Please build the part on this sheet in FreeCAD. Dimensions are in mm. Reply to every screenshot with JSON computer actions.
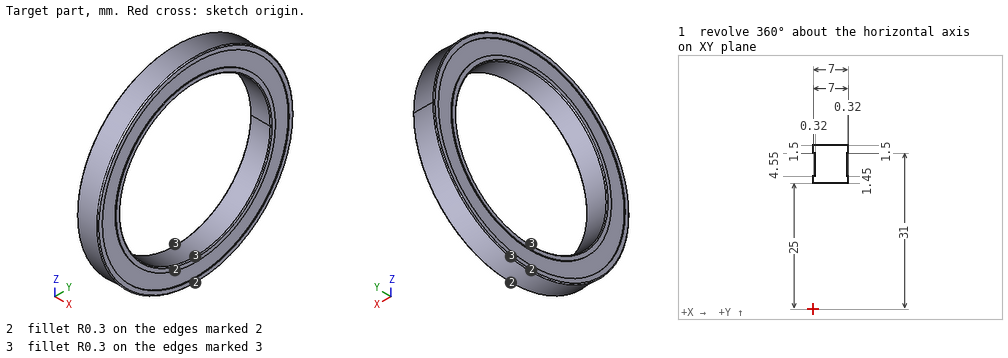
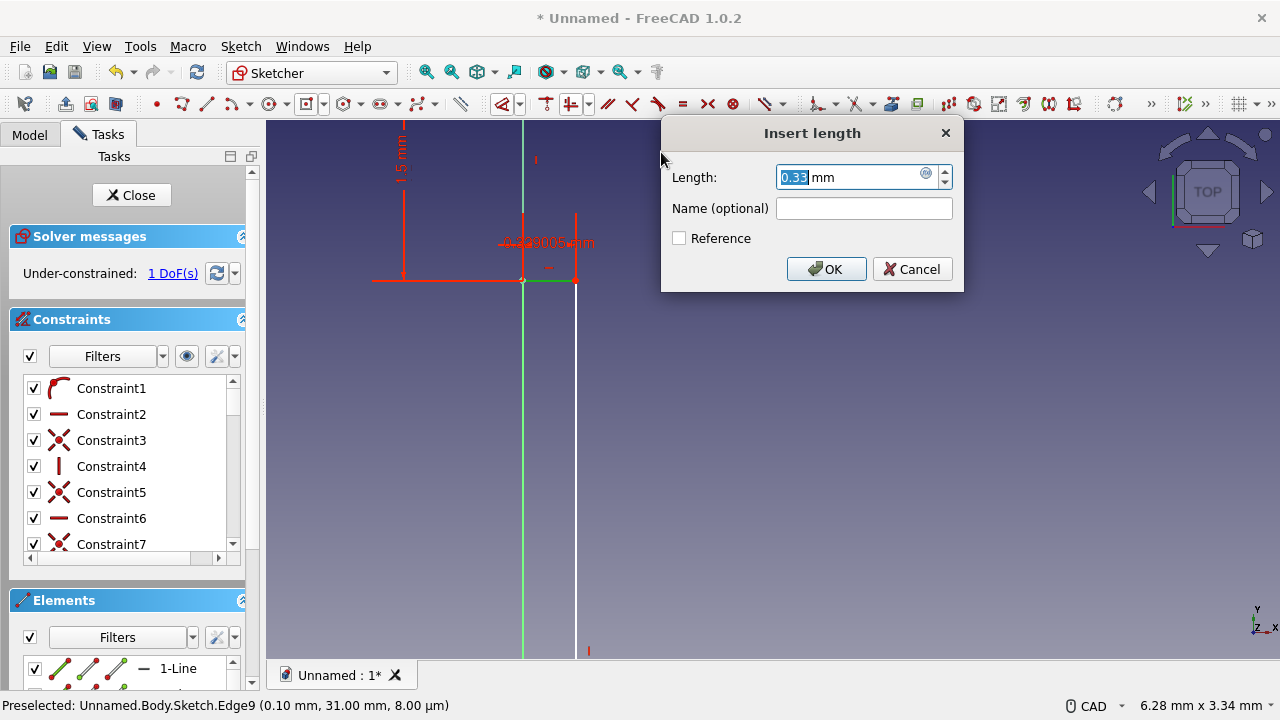
{"action": "type", "text": "0.32"}
{"action": "key", "text": "Return"}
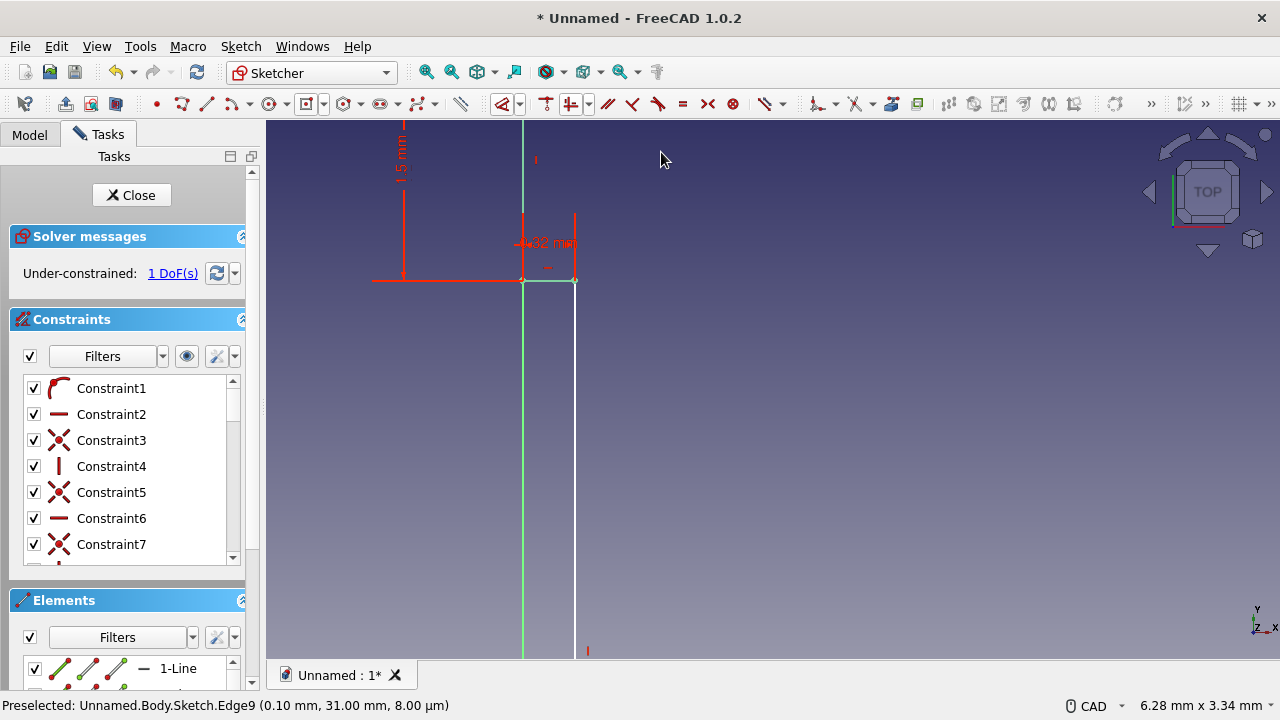
{"action": "left_click", "coordinate": [575, 502]}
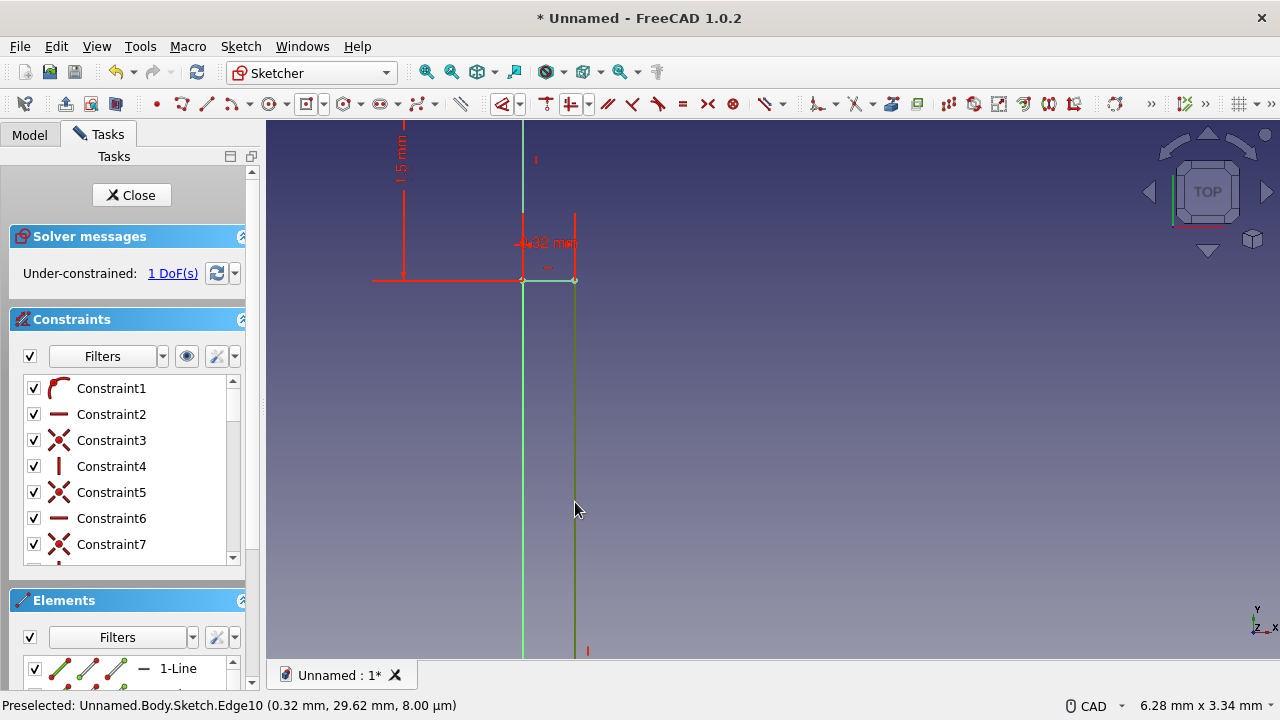
{"action": "key", "text": "i"}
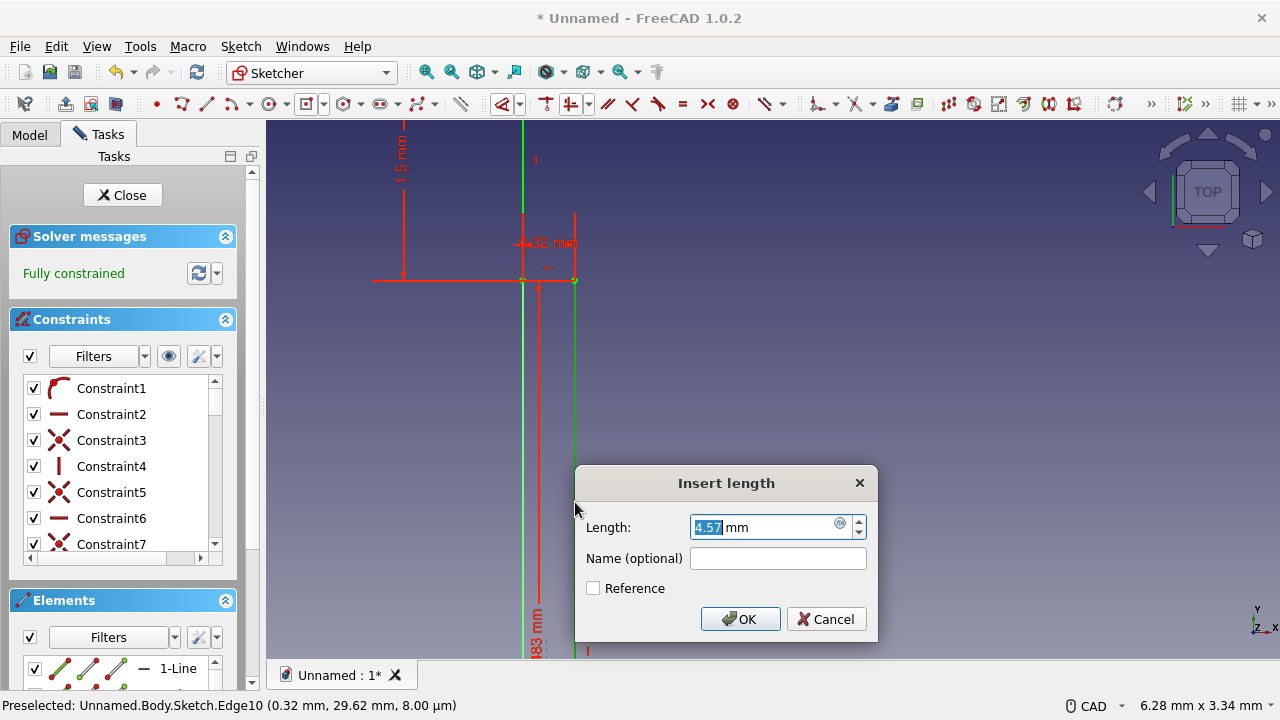
{"action": "type", "text": "4.55"}
{"action": "key", "text": "Return"}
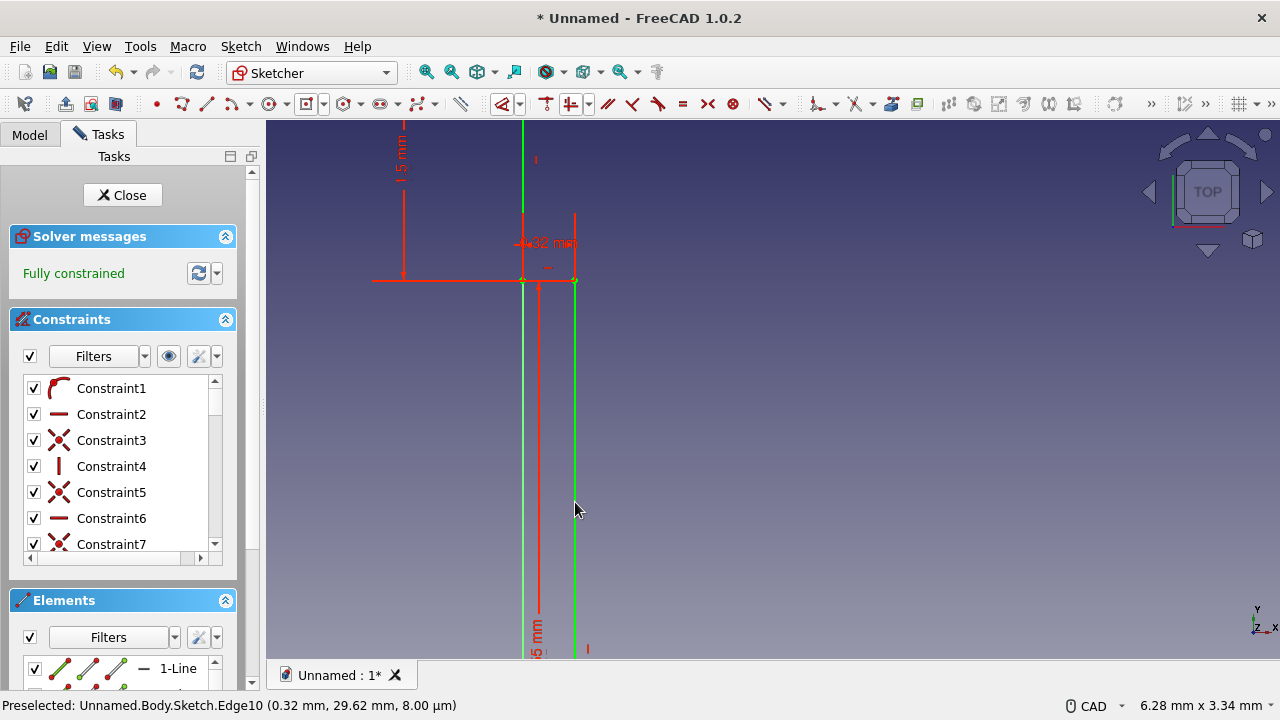
{"action": "left_click", "coordinate": [123, 195]}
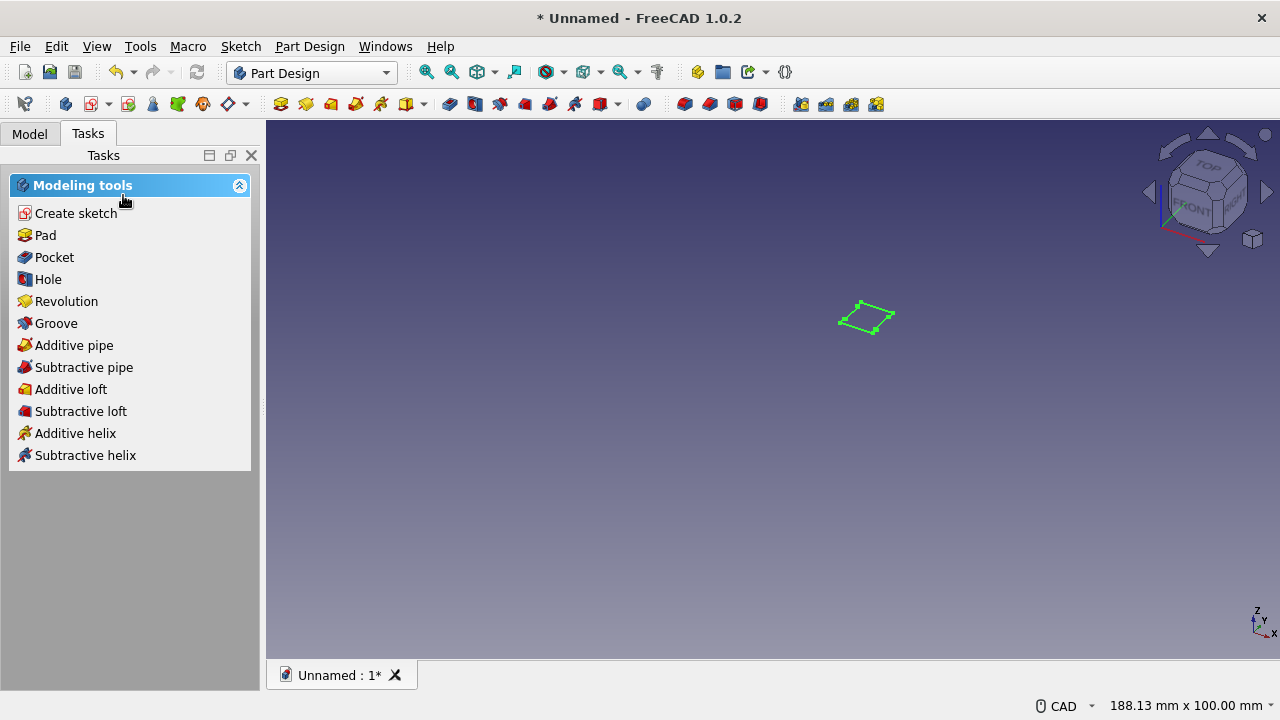
{"action": "left_click", "coordinate": [306, 104]}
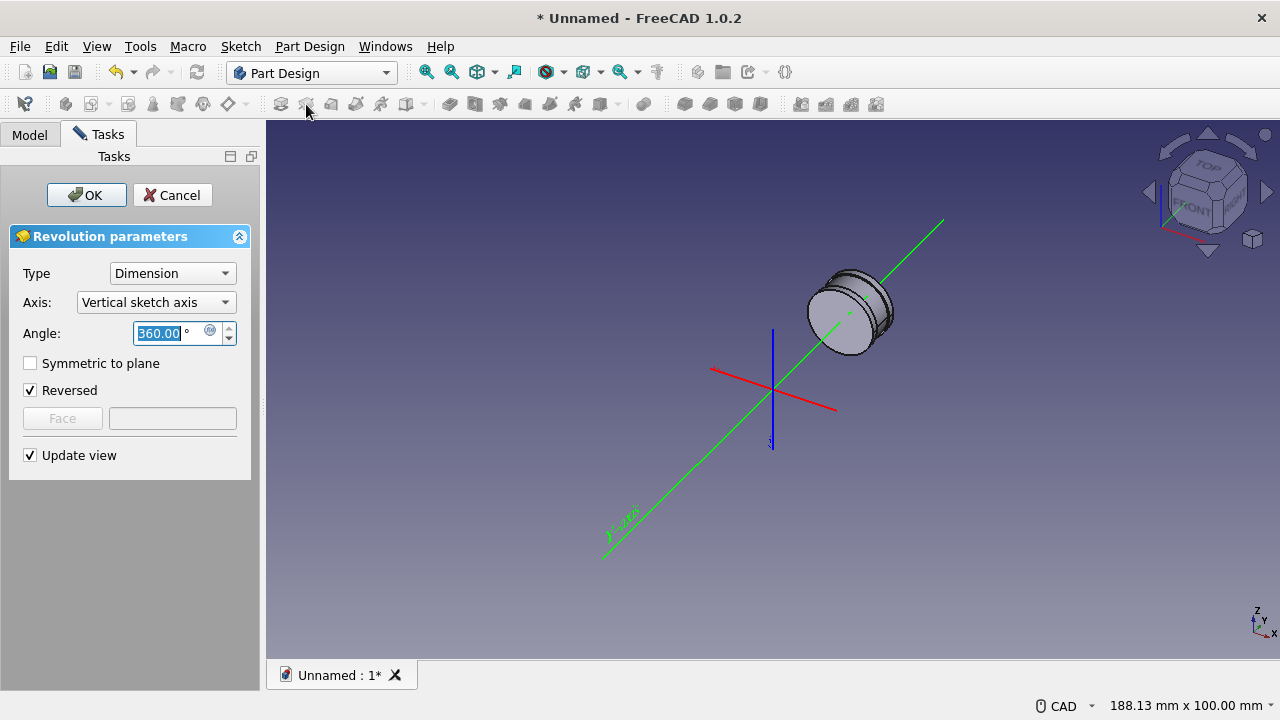
{"action": "left_click", "coordinate": [157, 302]}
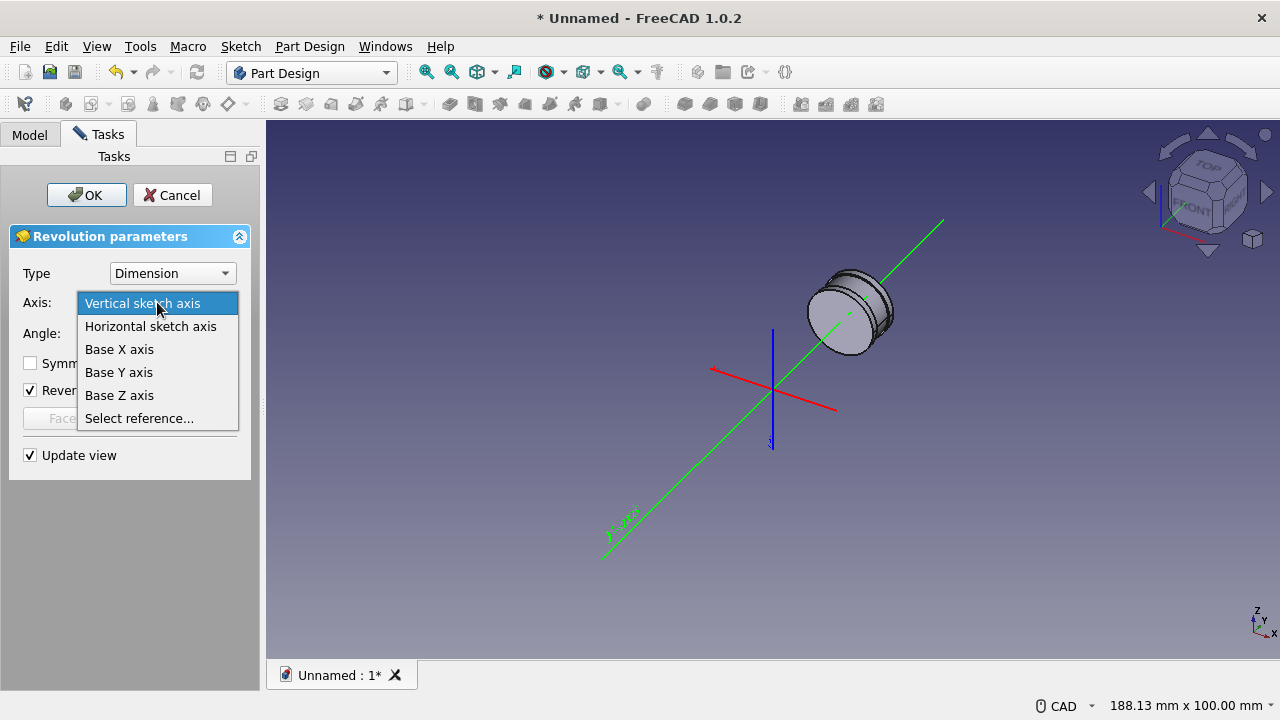
{"action": "left_click", "coordinate": [156, 326]}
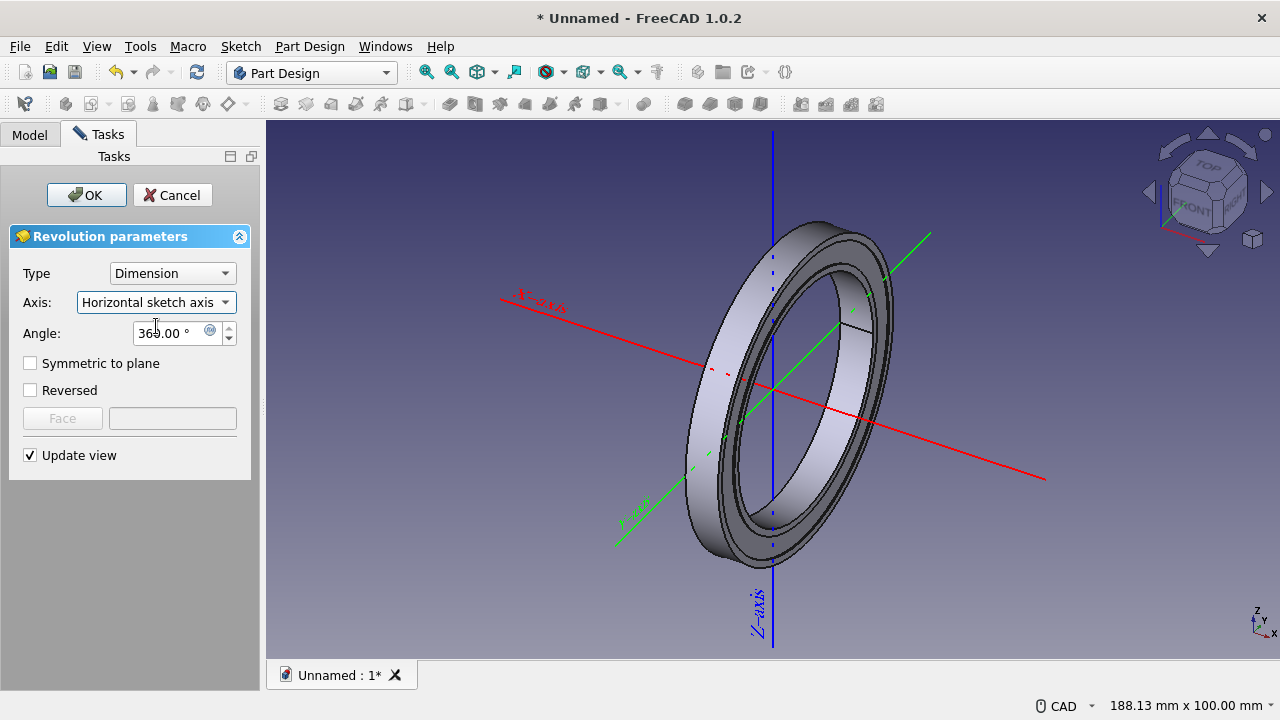
{"action": "left_click", "coordinate": [87, 195]}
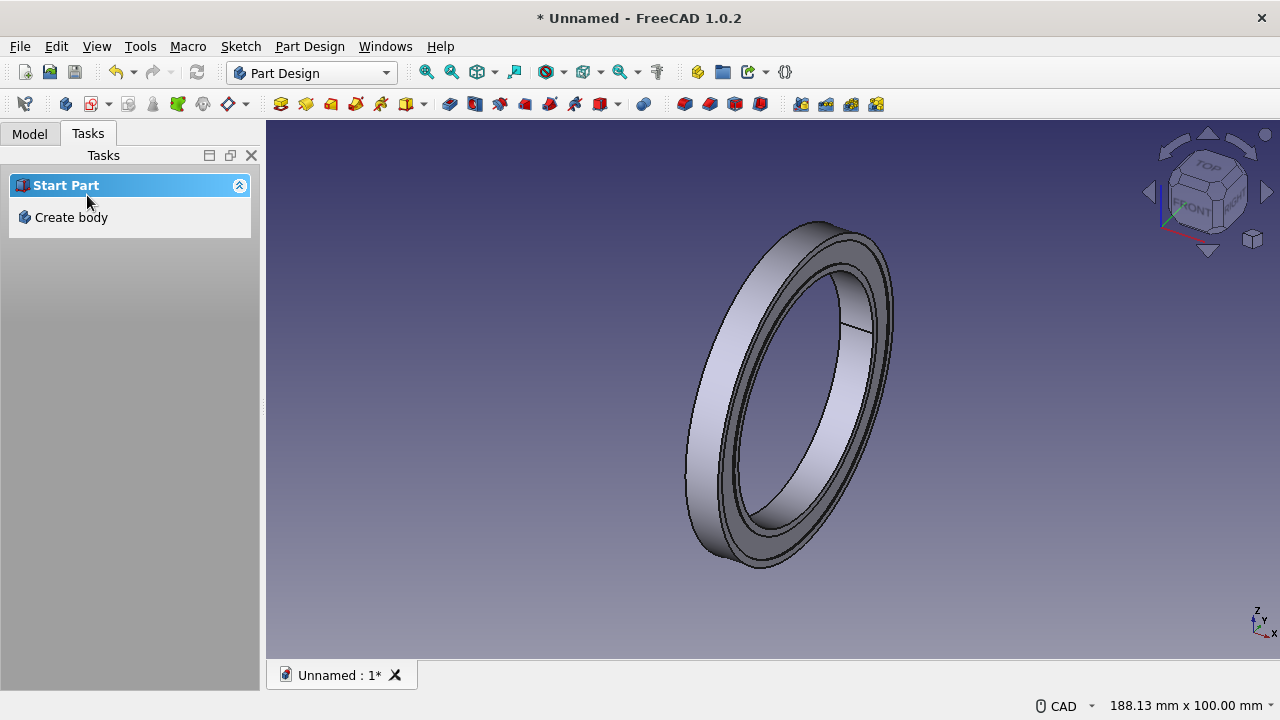
{"action": "left_click", "coordinate": [718, 486]}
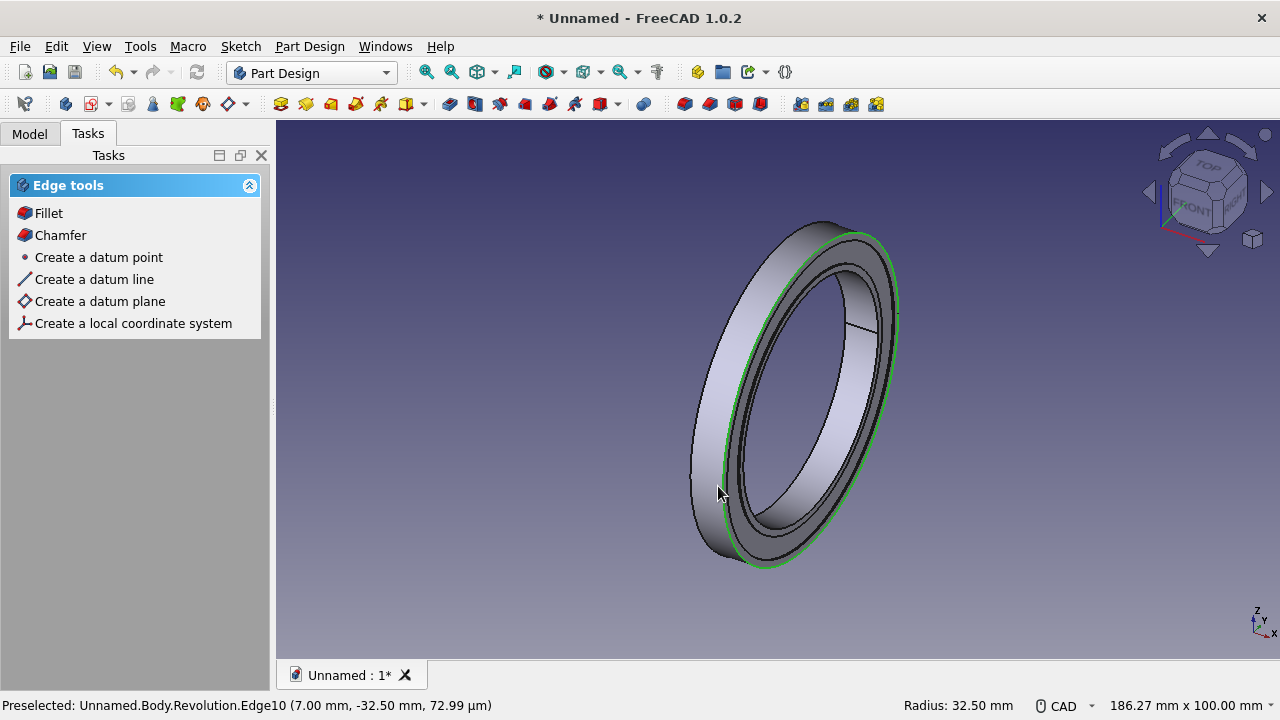
{"action": "key", "text": "0"}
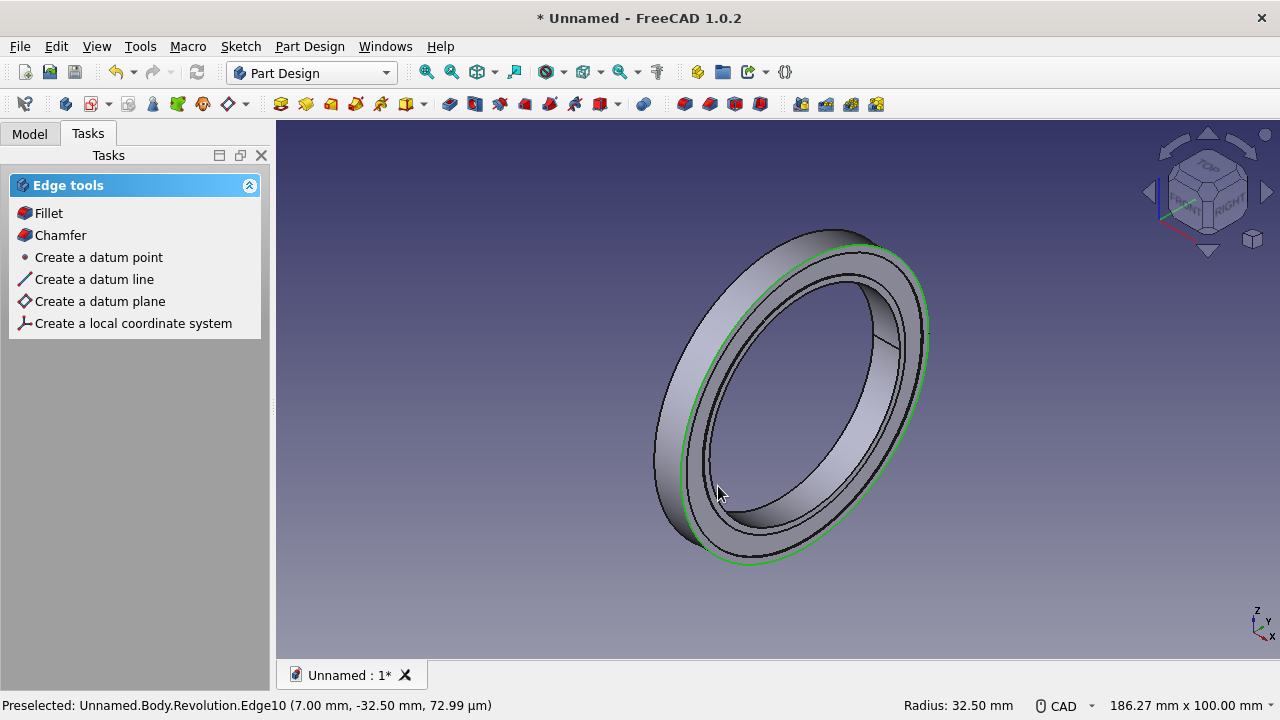
{"action": "key", "text": "2"}